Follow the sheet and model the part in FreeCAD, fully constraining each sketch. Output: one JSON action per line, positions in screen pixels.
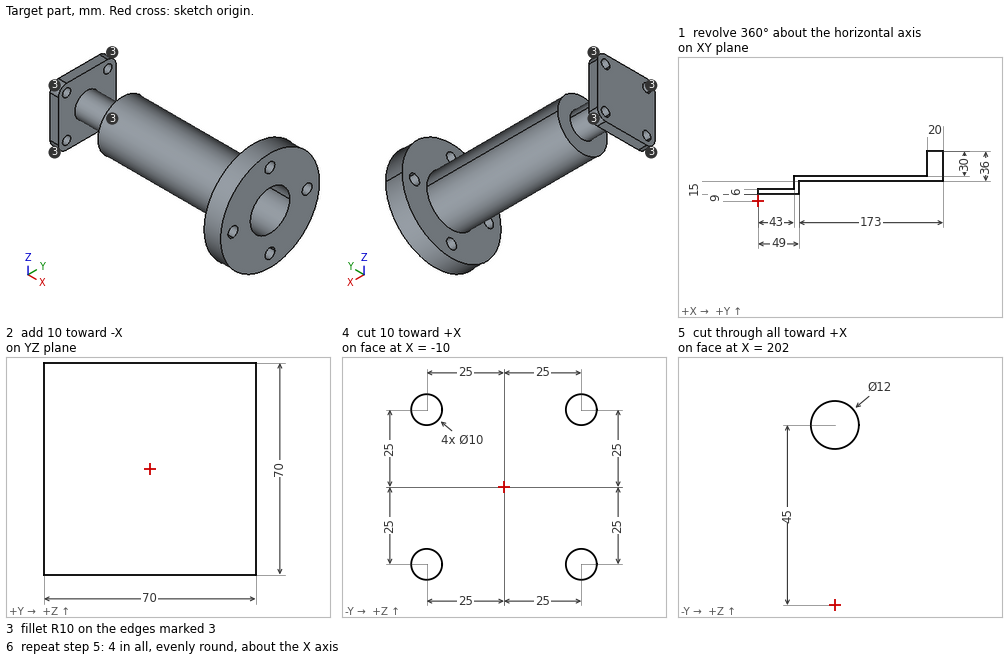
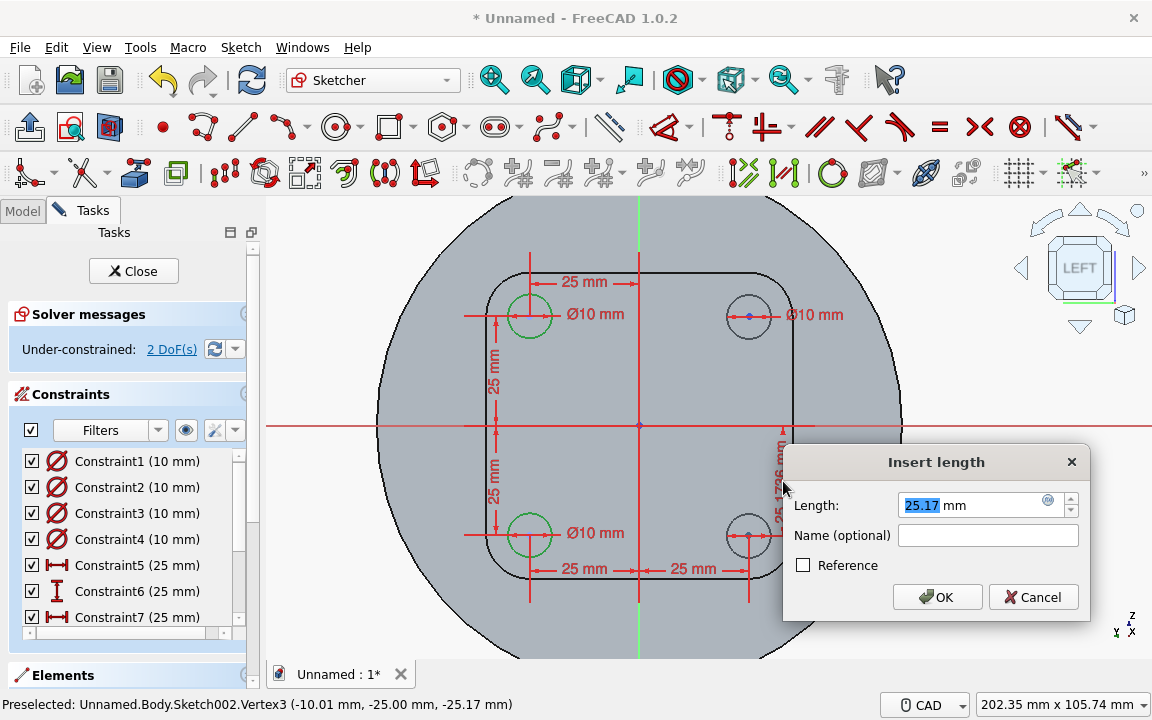
{"action": "type", "text": "25"}
{"action": "key", "text": "Return"}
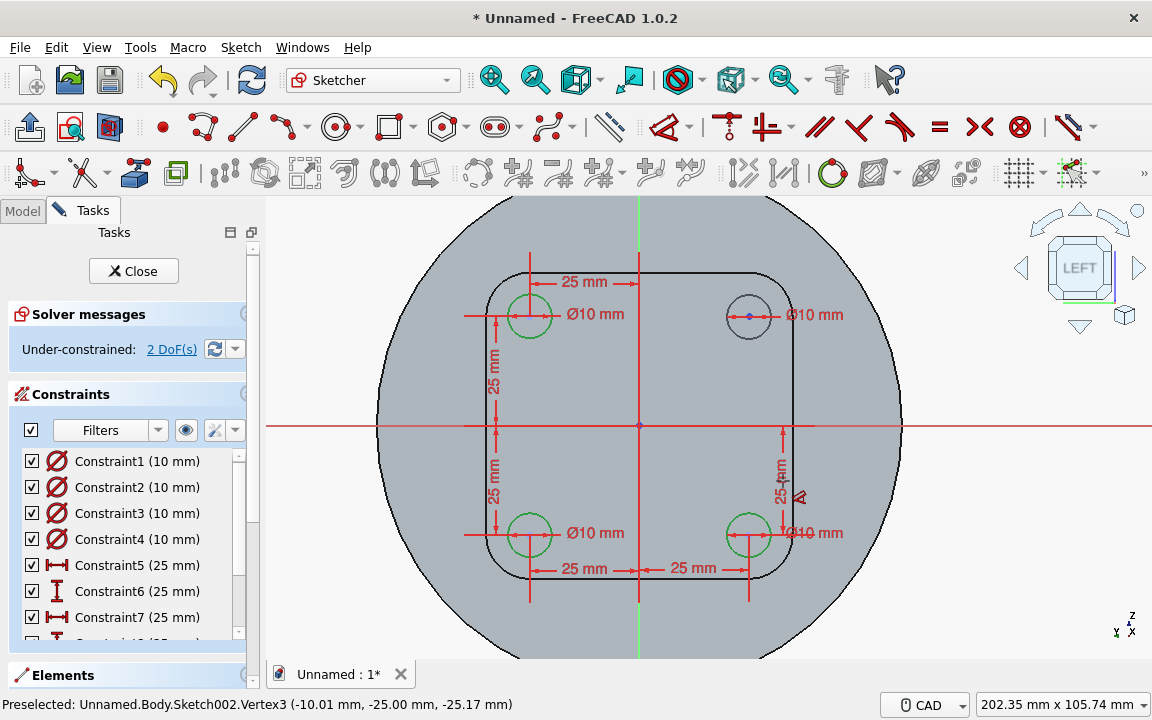
{"action": "left_click", "coordinate": [749, 317]}
{"action": "left_click", "coordinate": [694, 283]}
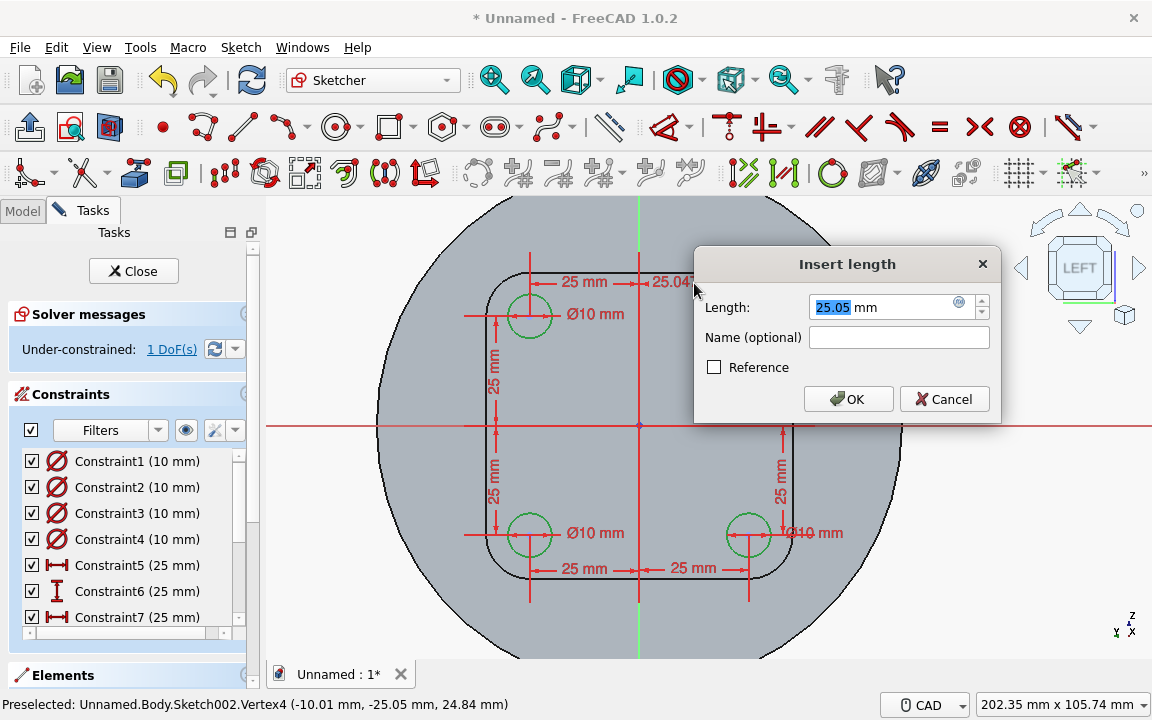
{"action": "type", "text": "25"}
{"action": "key", "text": "Return"}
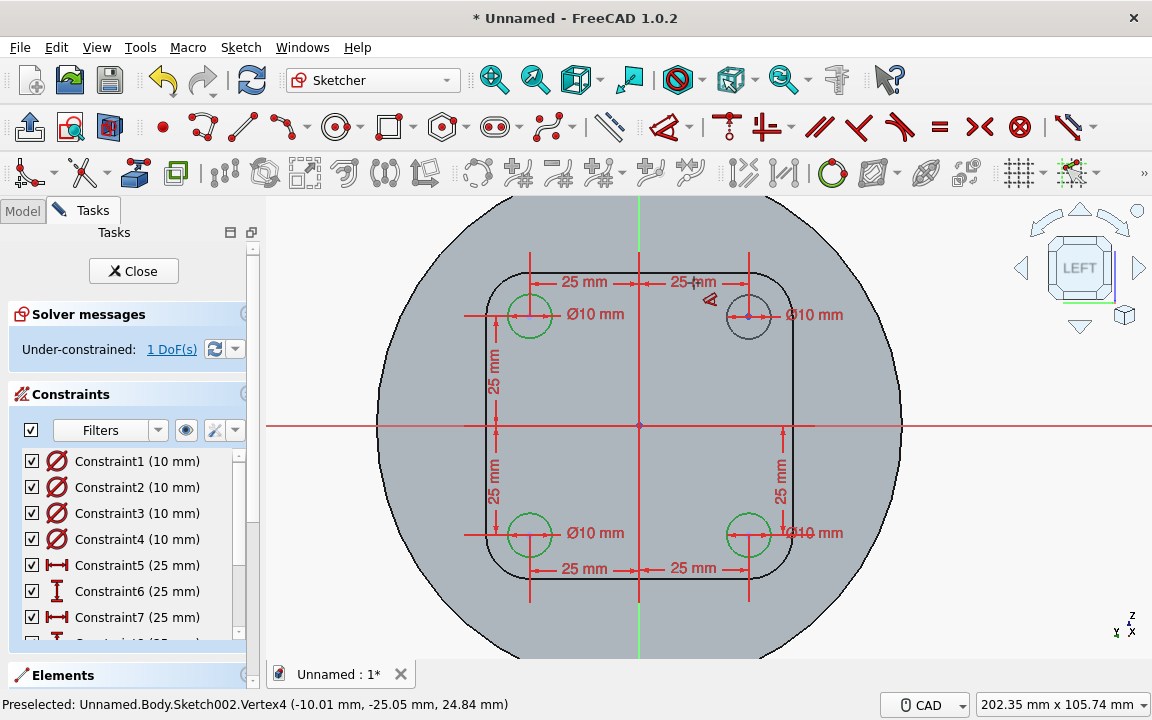
{"action": "left_click", "coordinate": [749, 317]}
{"action": "left_click", "coordinate": [783, 371]}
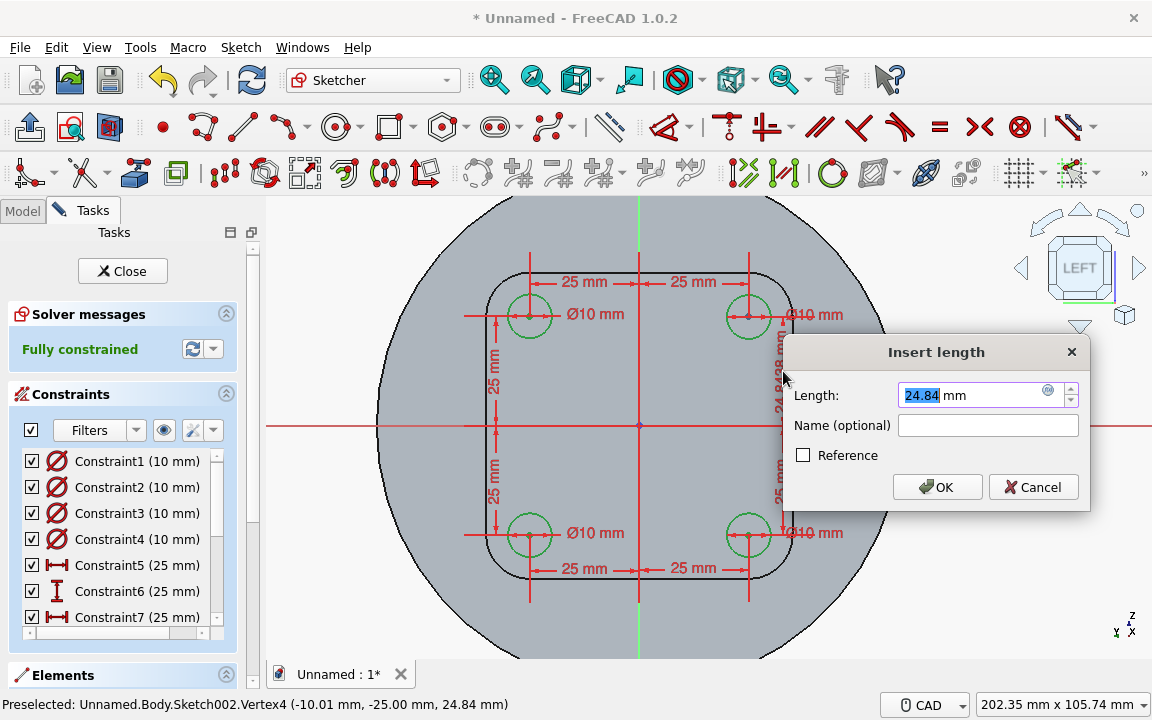
{"action": "type", "text": "25"}
{"action": "key", "text": "Return"}
{"action": "key", "text": "Escape"}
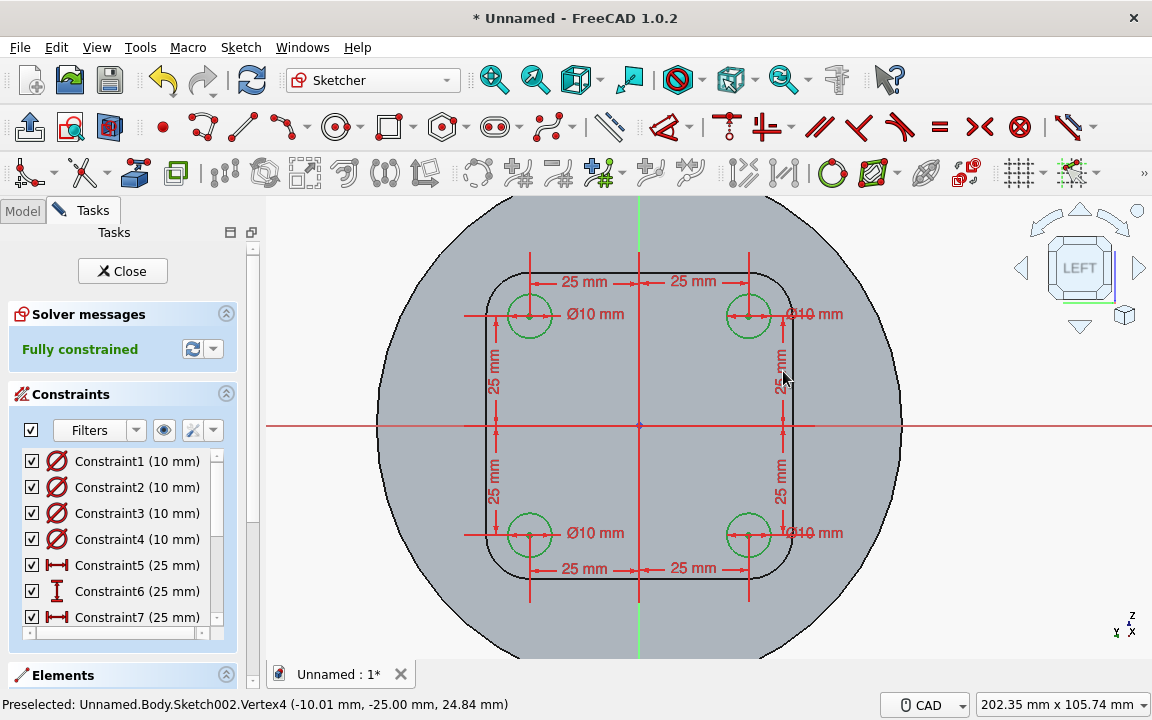
{"action": "left_click", "coordinate": [123, 271]}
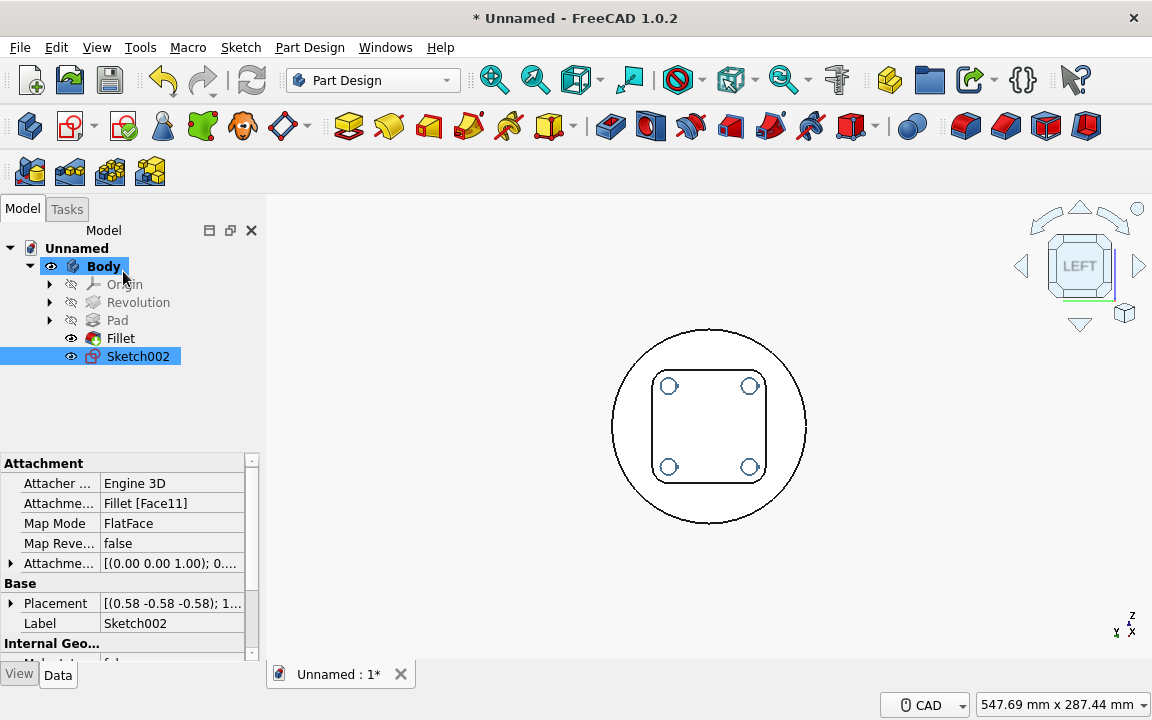
{"action": "left_click", "coordinate": [612, 126]}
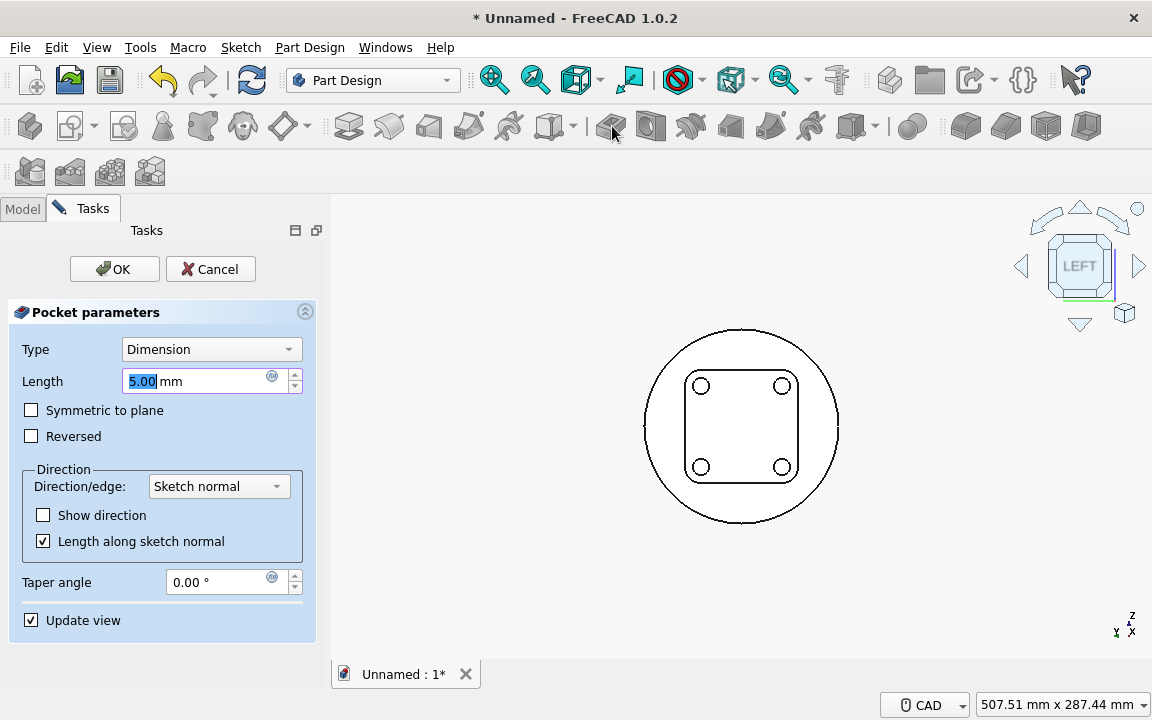
{"action": "type", "text": "10"}
{"action": "key", "text": "Tab"}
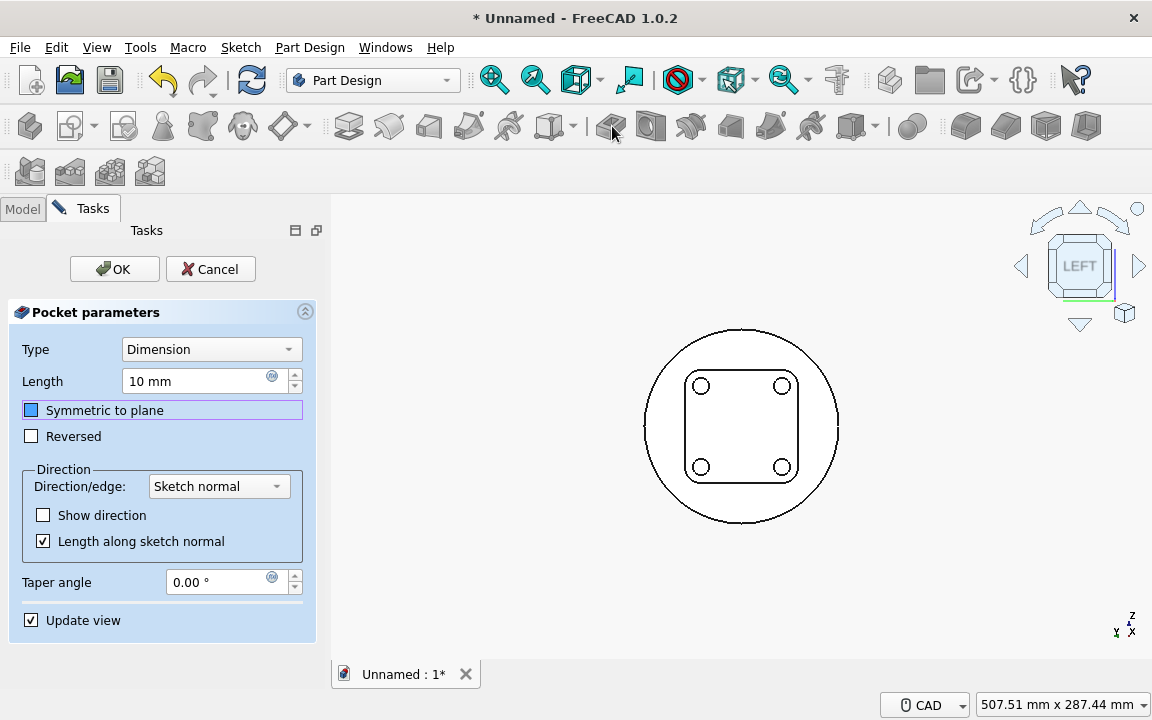
{"action": "left_click", "coordinate": [115, 269]}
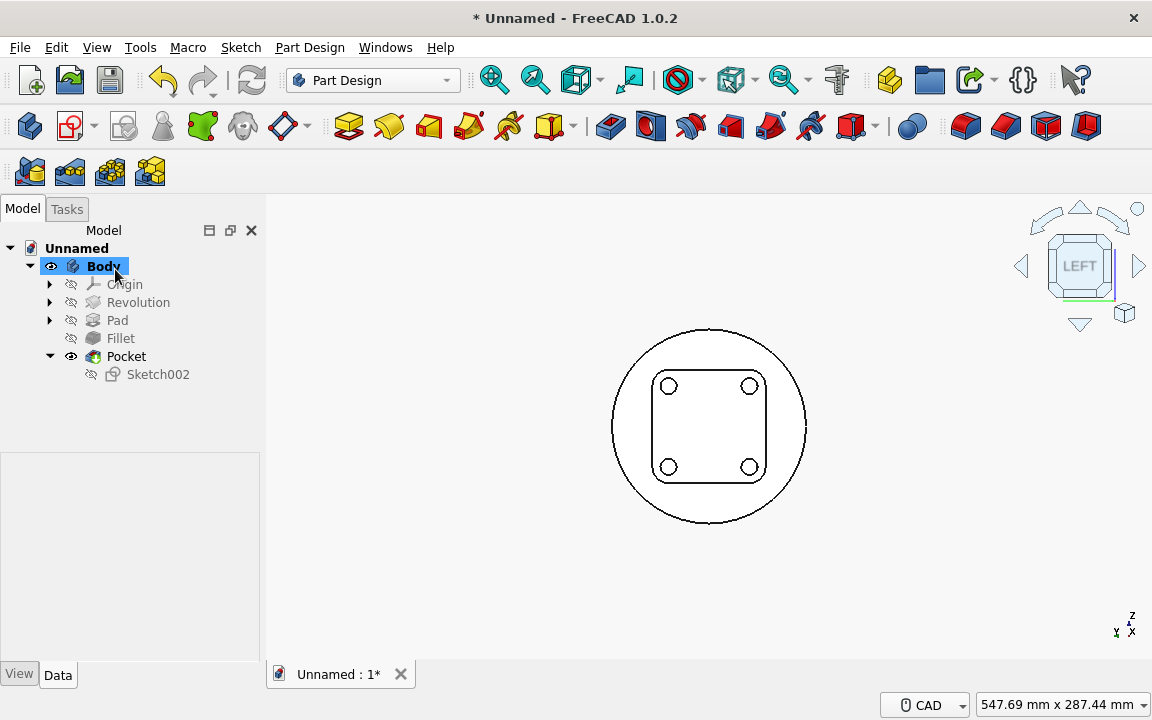
{"action": "left_click", "coordinate": [496, 80]}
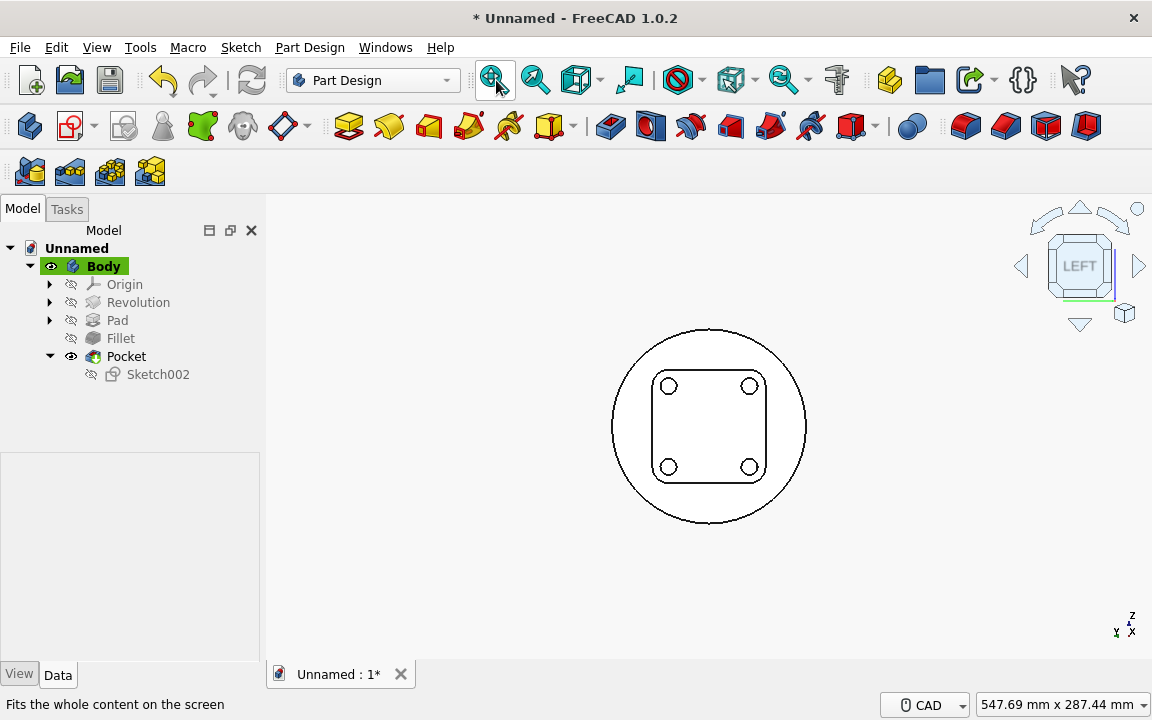
{"action": "left_click", "coordinate": [626, 425]}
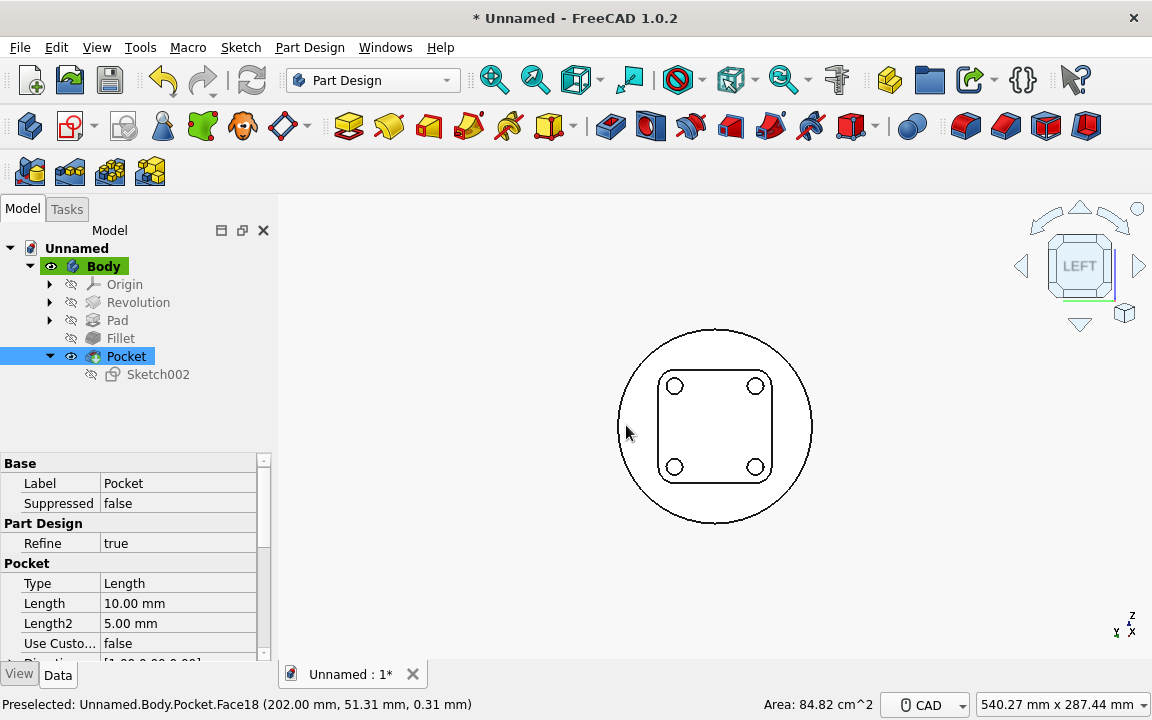
{"action": "left_click", "coordinate": [70, 126]}